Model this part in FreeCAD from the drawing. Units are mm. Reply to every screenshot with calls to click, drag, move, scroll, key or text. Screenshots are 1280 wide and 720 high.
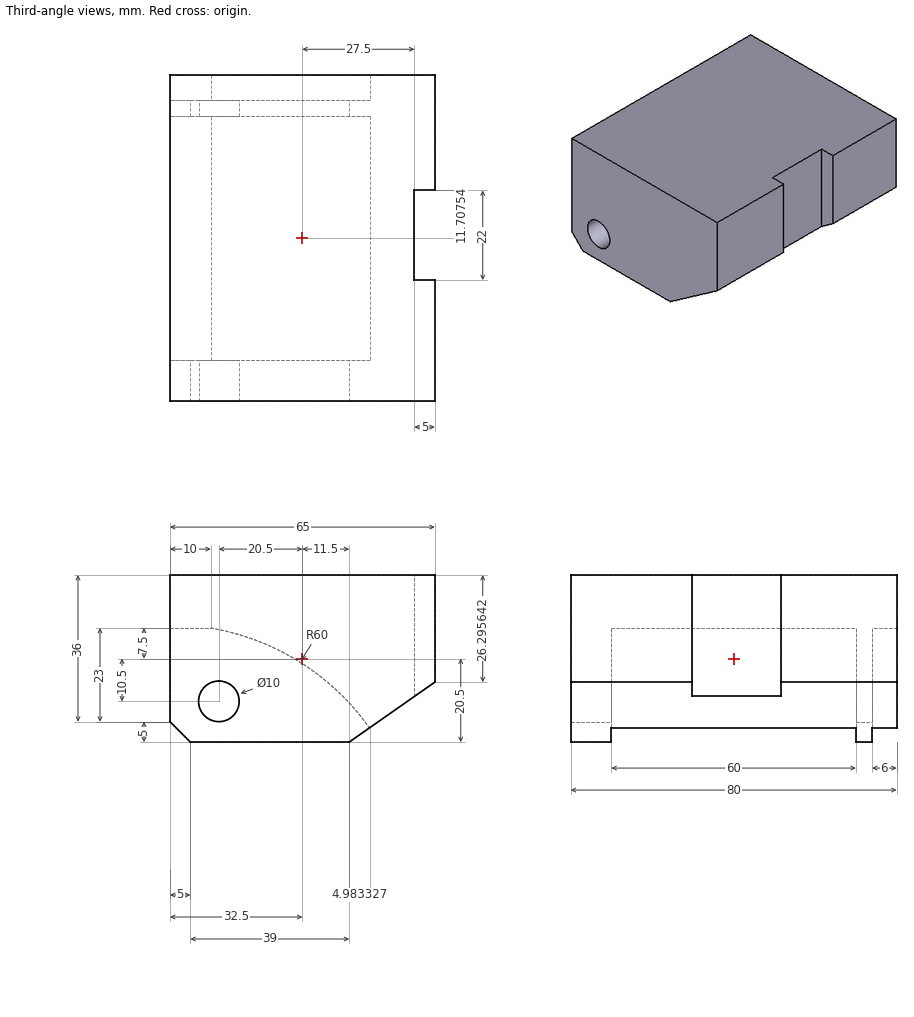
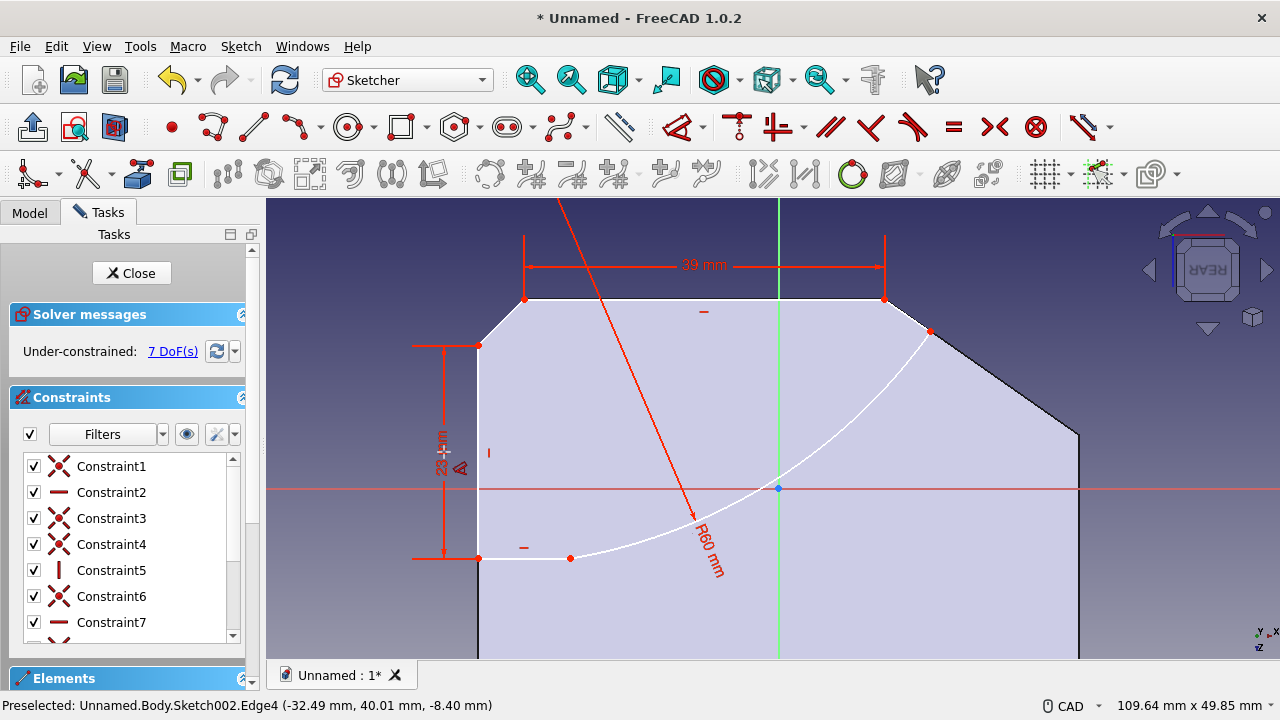
click(506, 559)
click(524, 593)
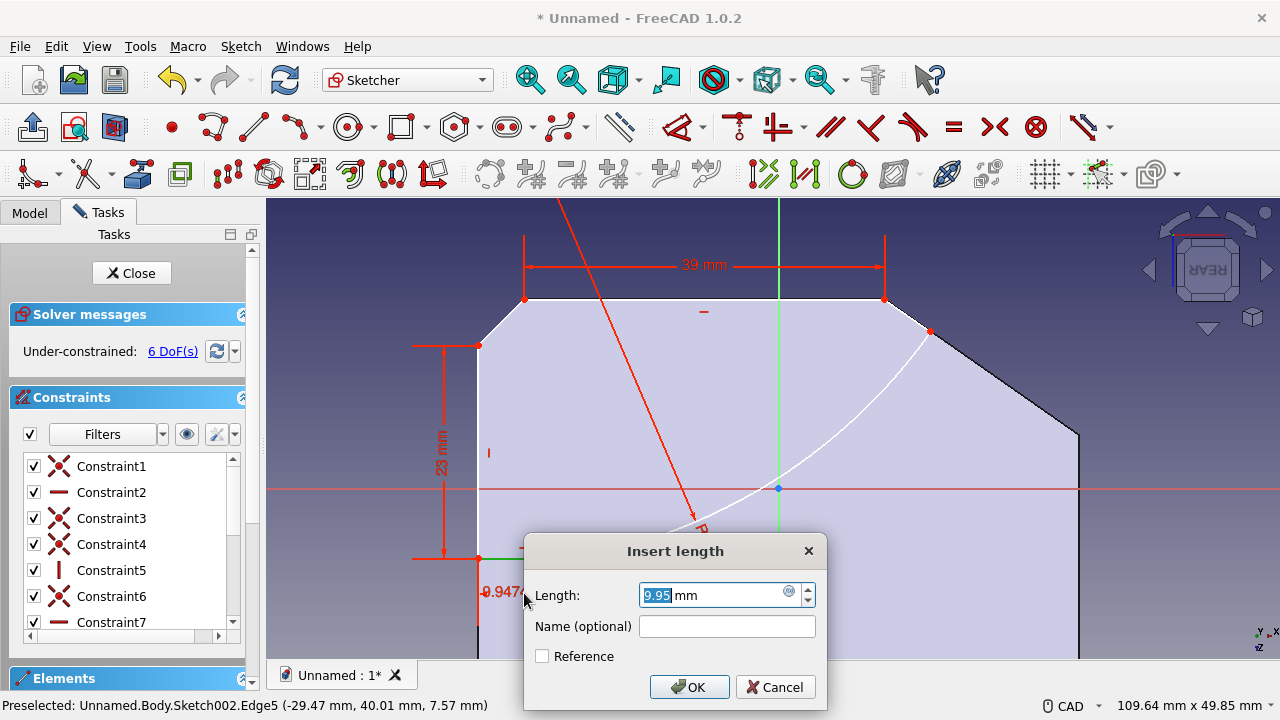
text(10)
key(Return)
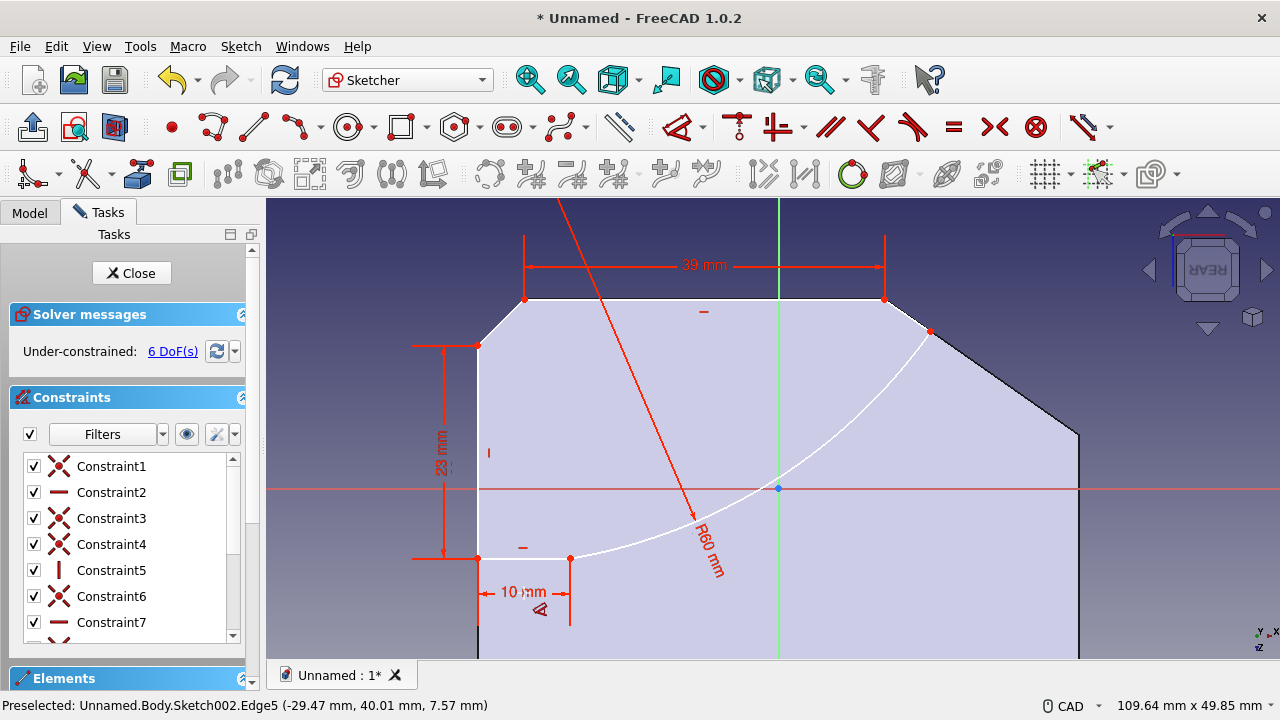
click(510, 314)
click(501, 266)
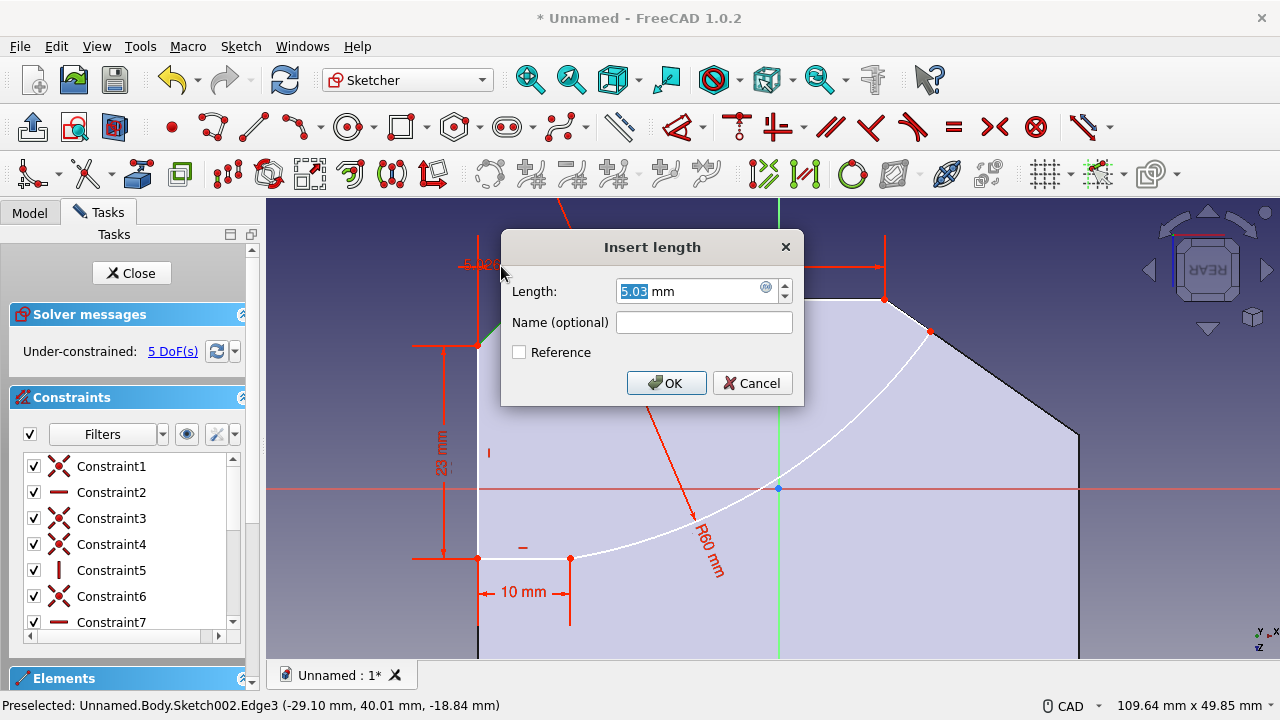
text(5)
key(Return)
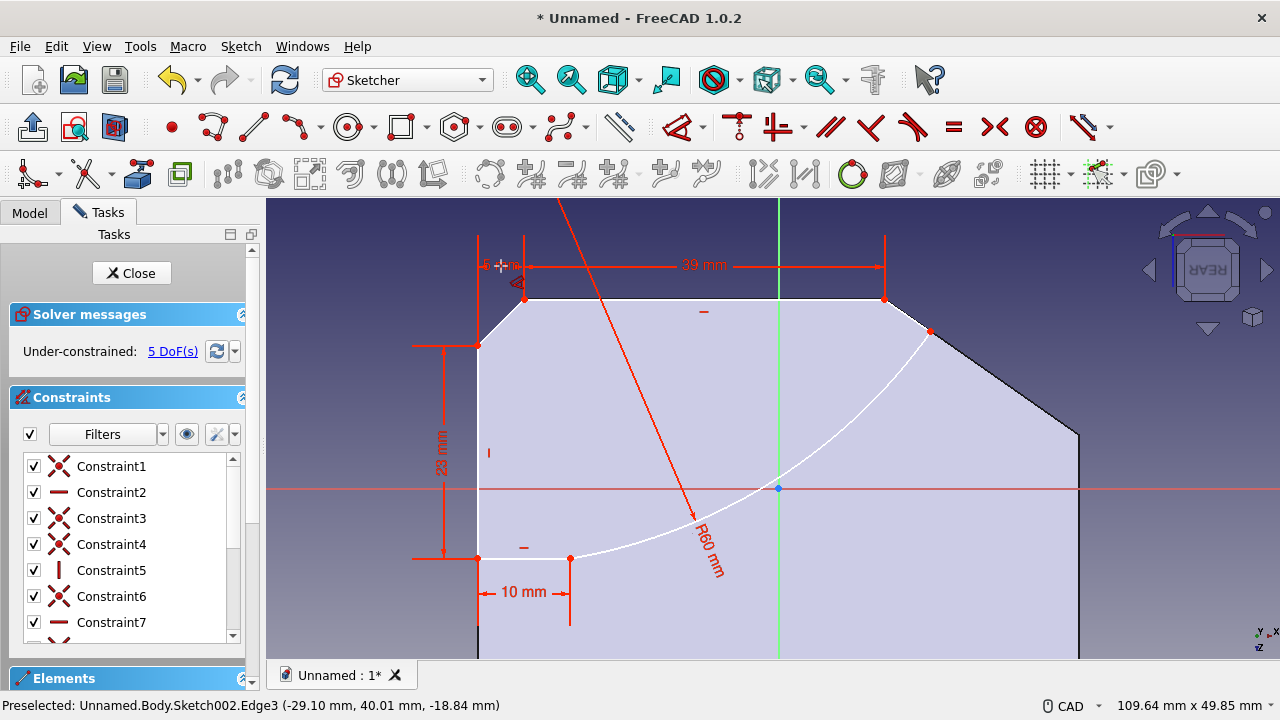
click(510, 314)
click(444, 323)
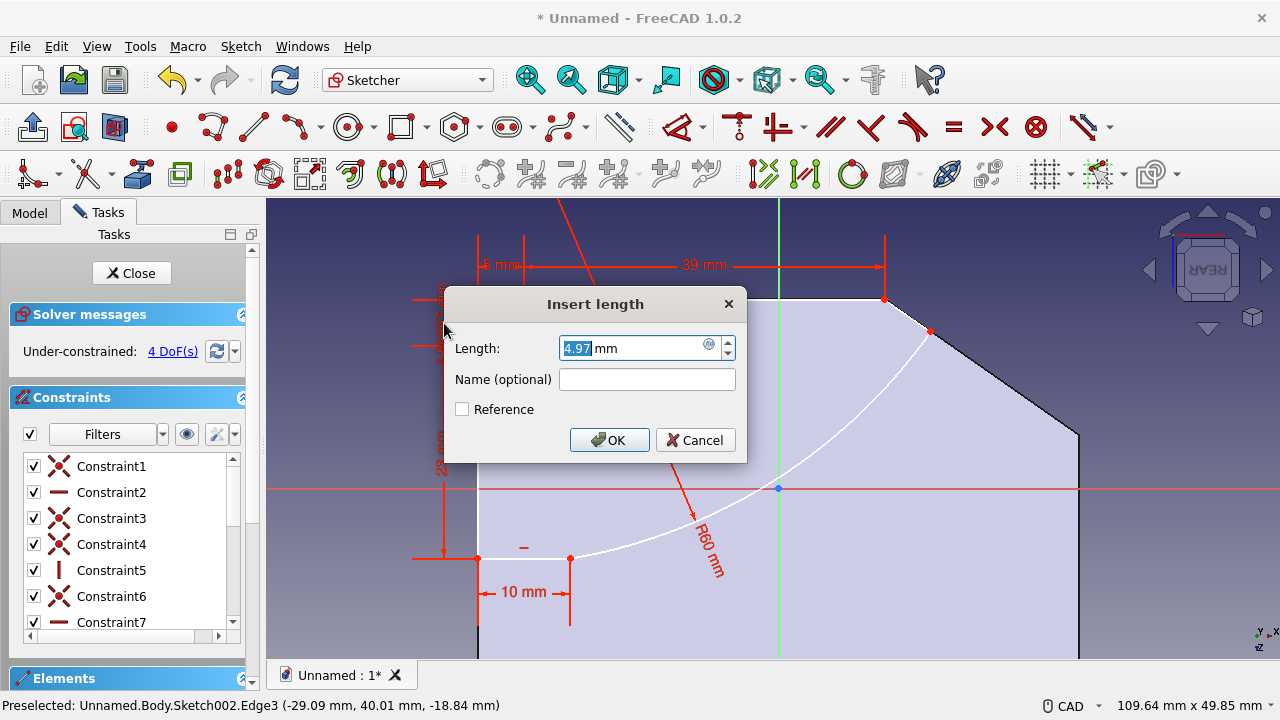
text(5)
key(Return)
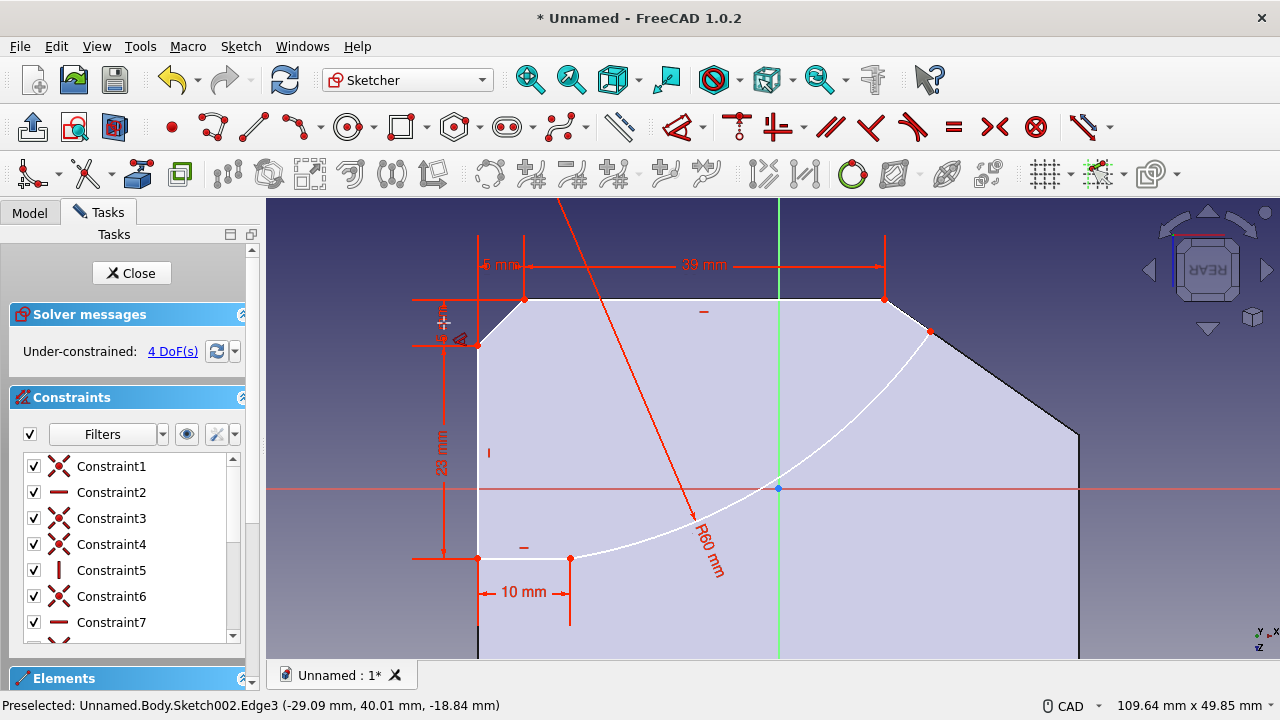
click(478, 559)
click(444, 524)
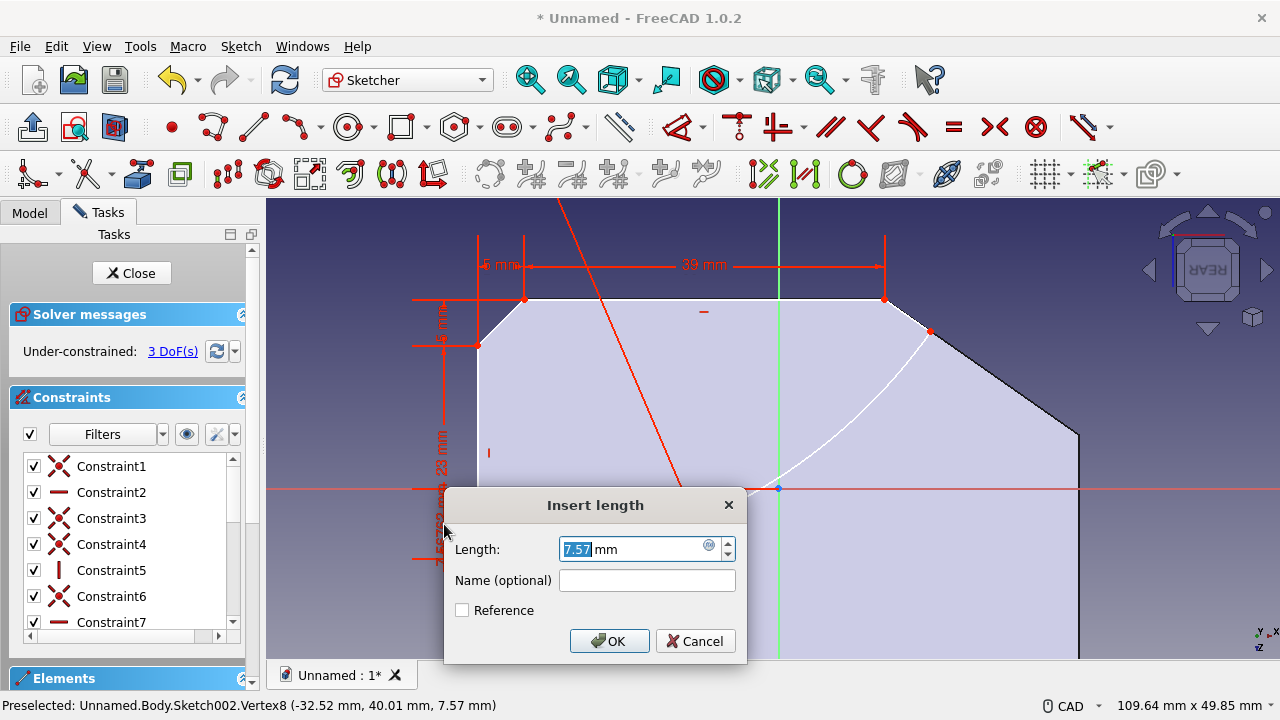
text(7.5)
key(Return)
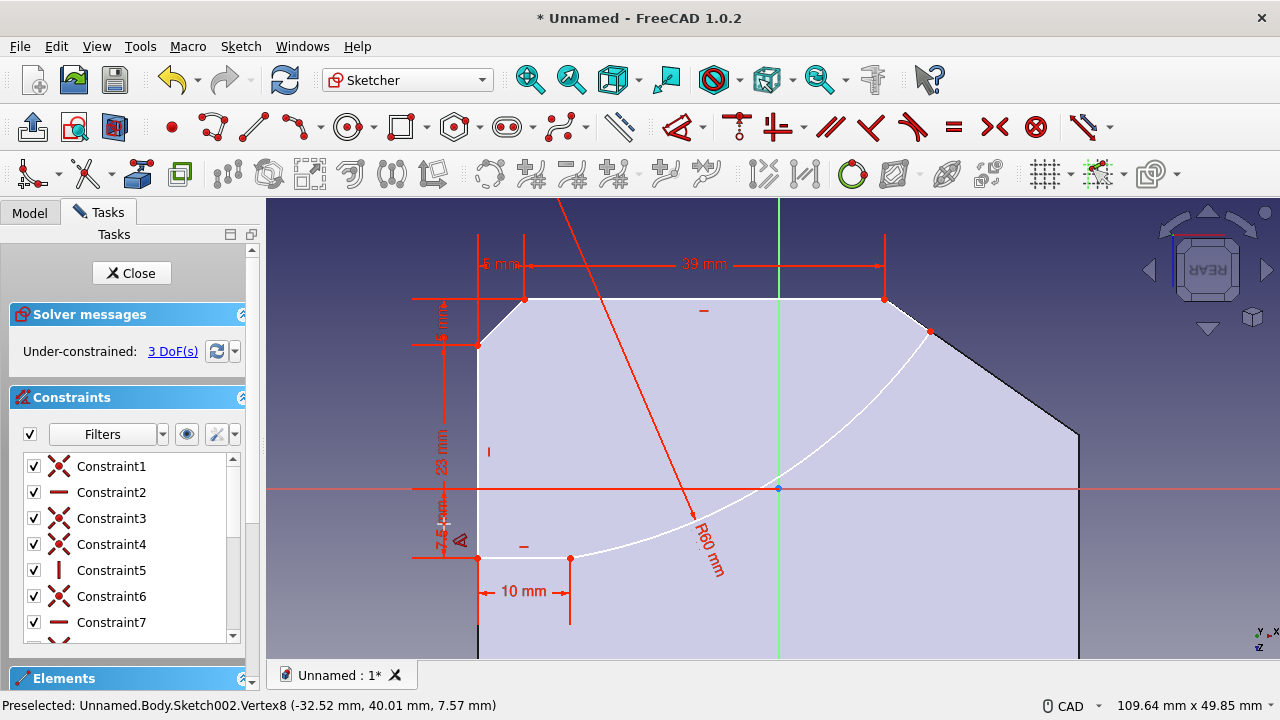
click(885, 299)
click(832, 265)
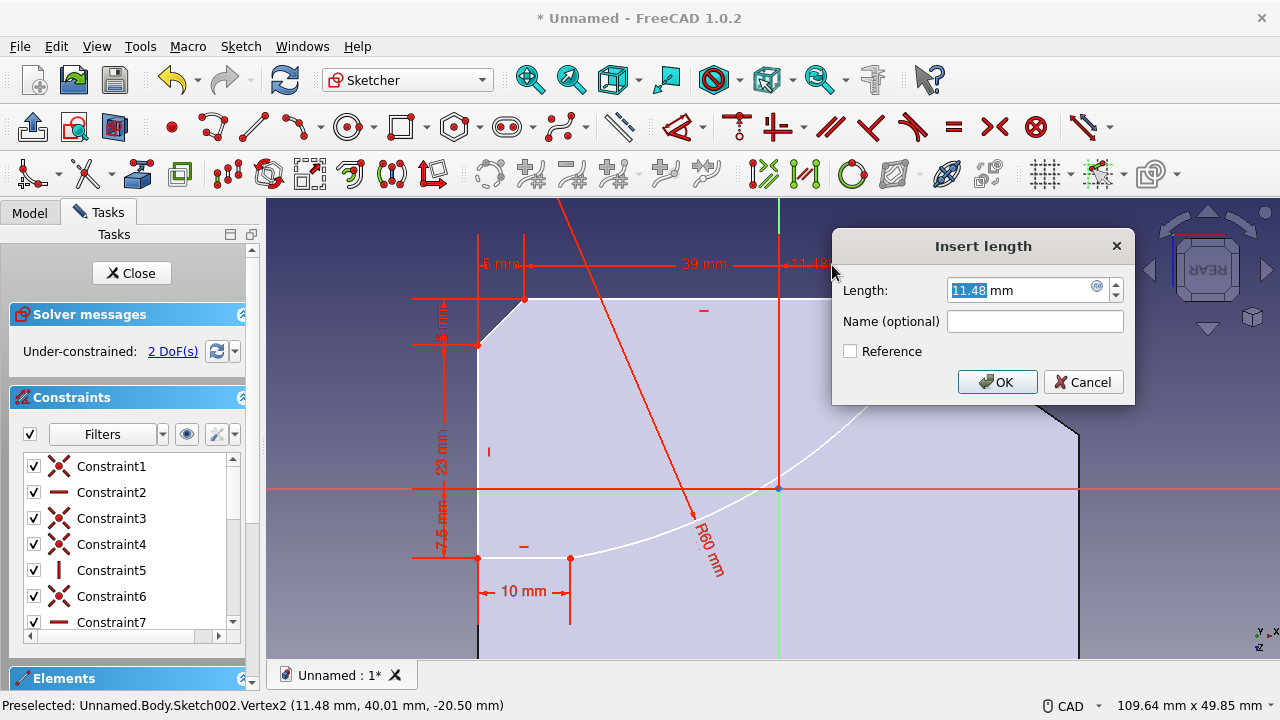
text(11.5)
key(Return)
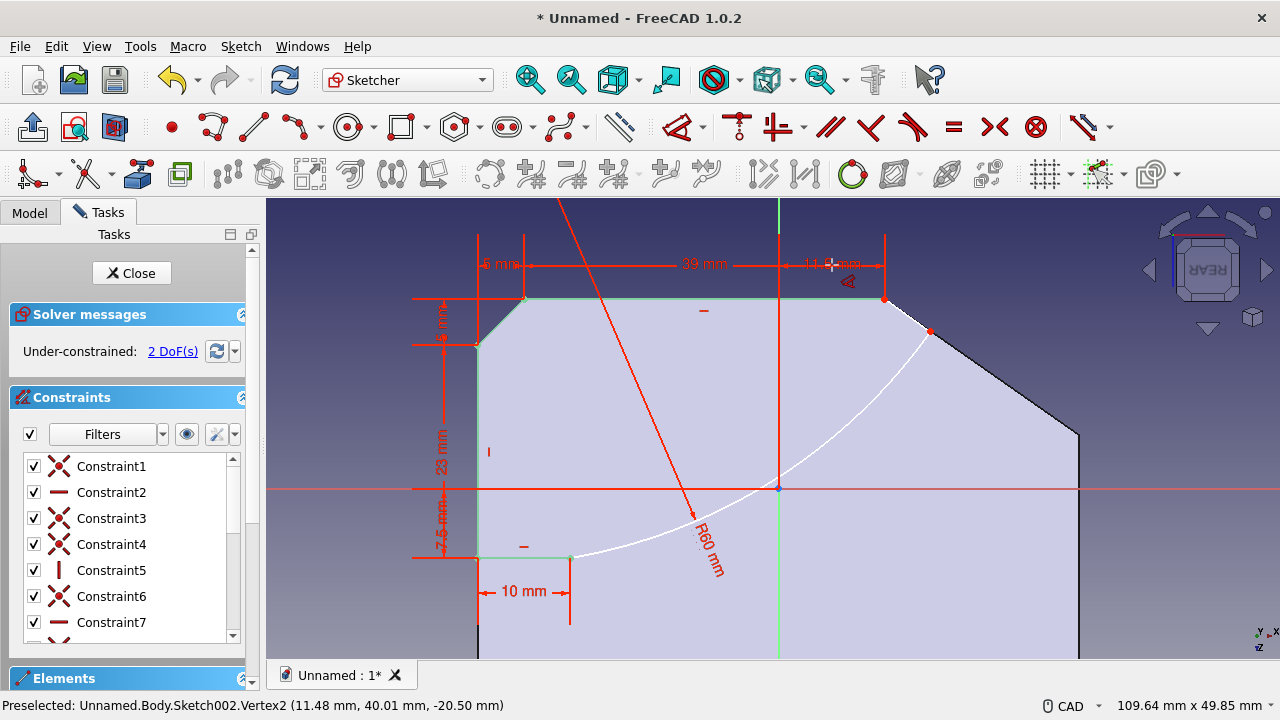
scroll(705, 604, down, 3)